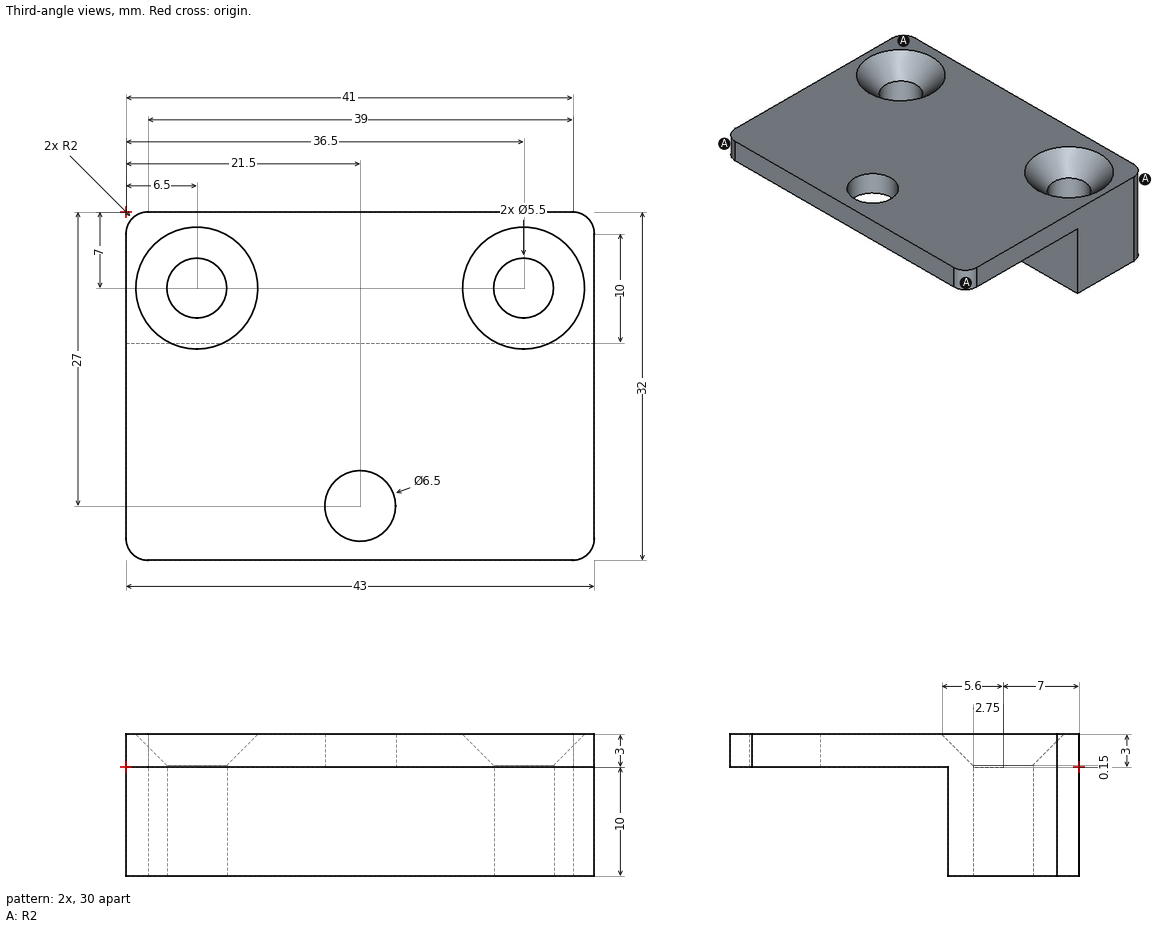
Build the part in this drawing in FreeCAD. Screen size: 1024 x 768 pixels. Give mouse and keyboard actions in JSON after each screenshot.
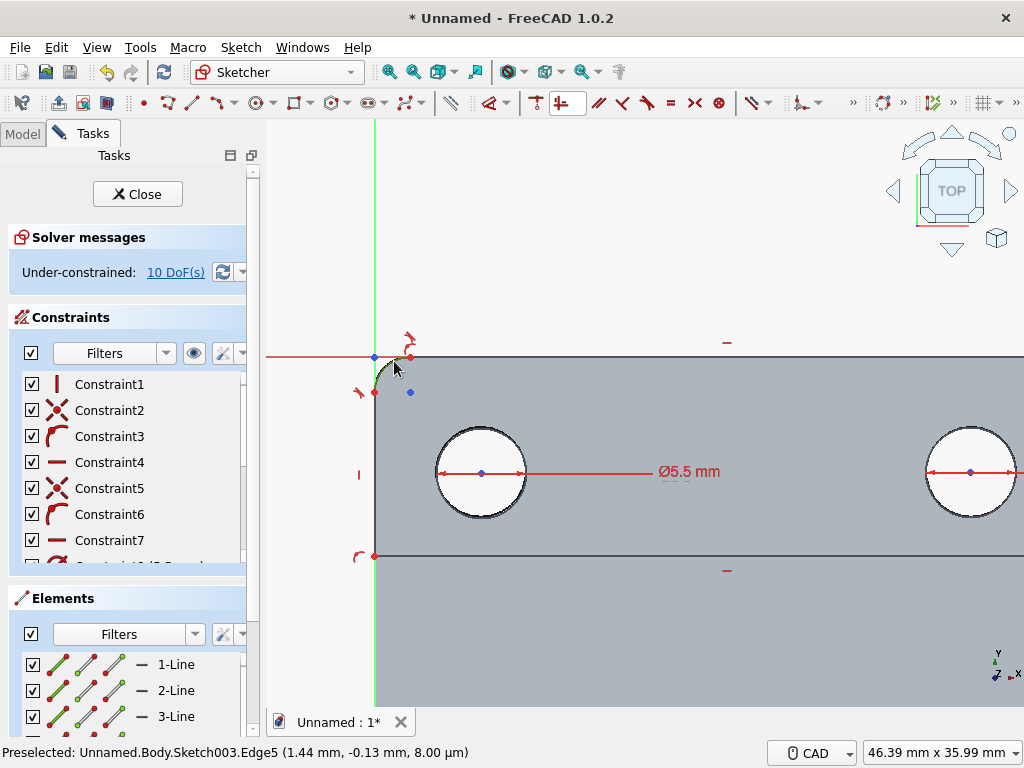
{"action": "scroll", "coordinate": [395, 361], "scroll_direction": "down", "scroll_amount": 3}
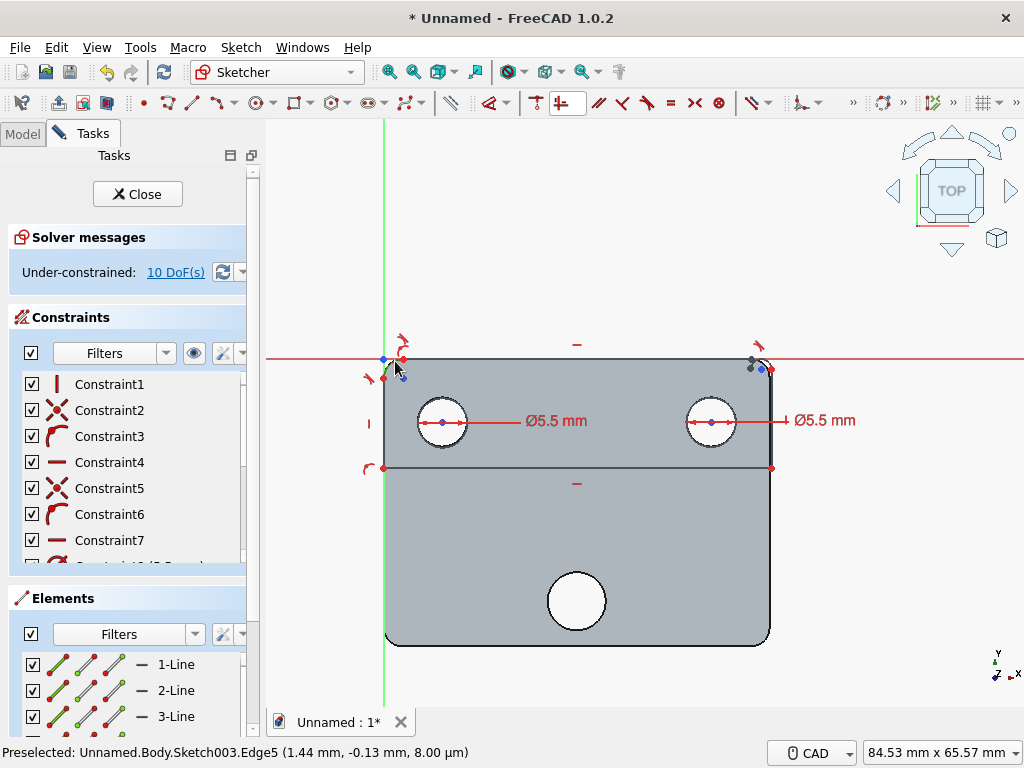
{"action": "scroll", "coordinate": [768, 361], "scroll_direction": "up", "scroll_amount": 2}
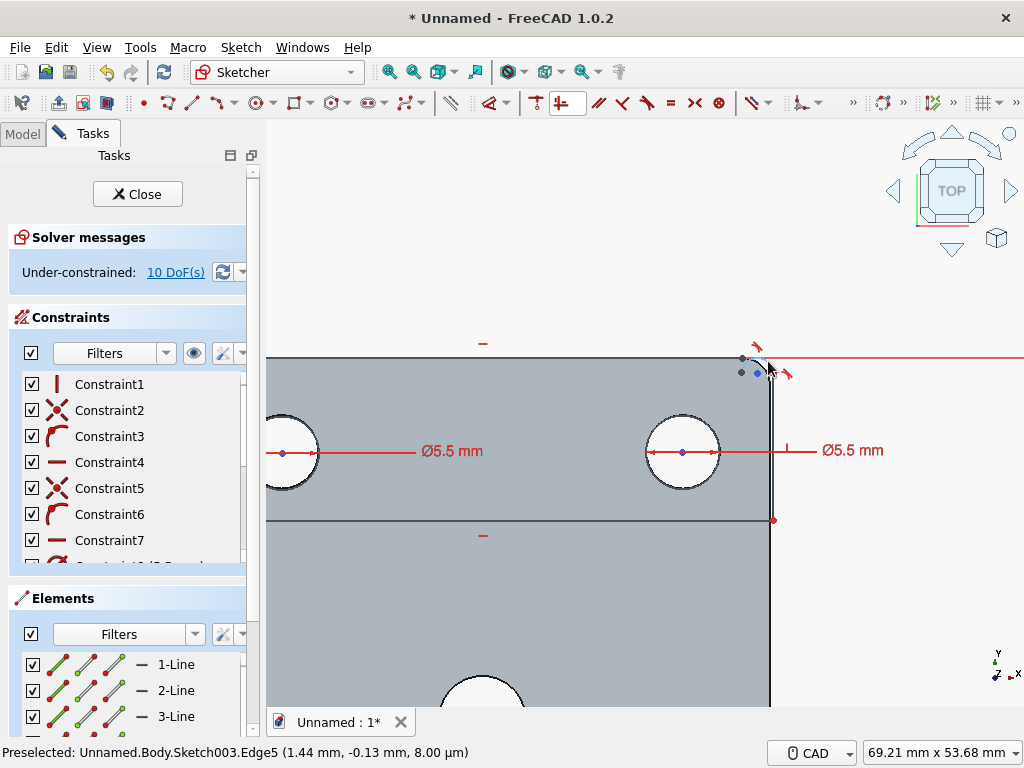
{"action": "left_click", "coordinate": [767, 361]}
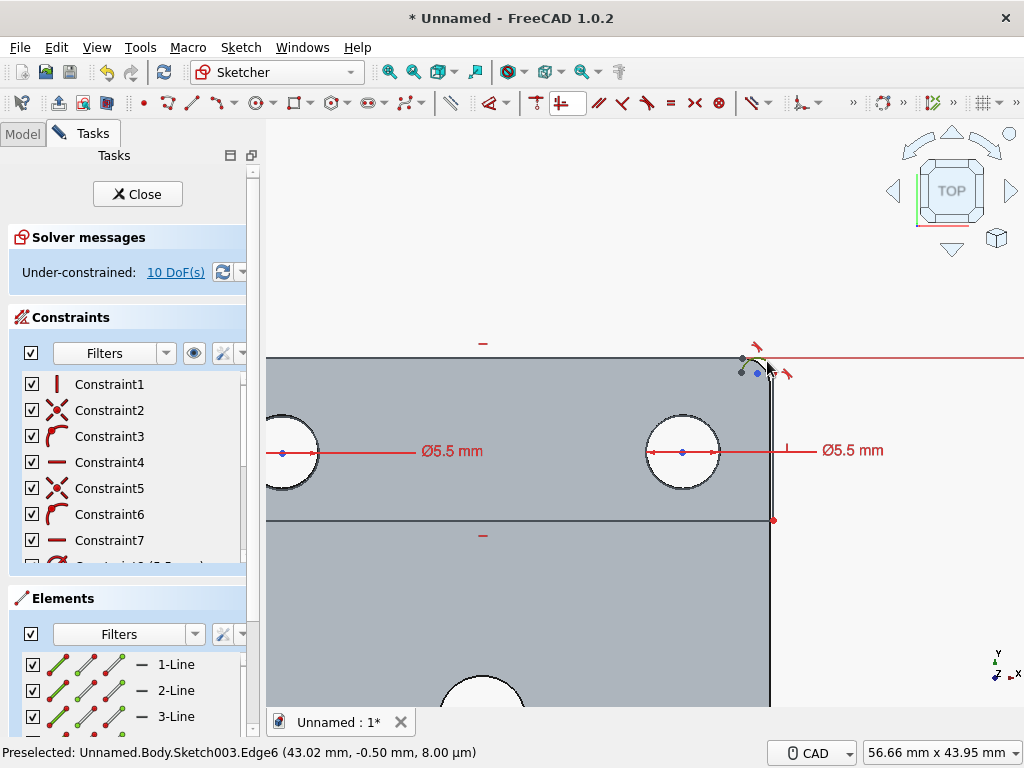
{"action": "key", "text": "e"}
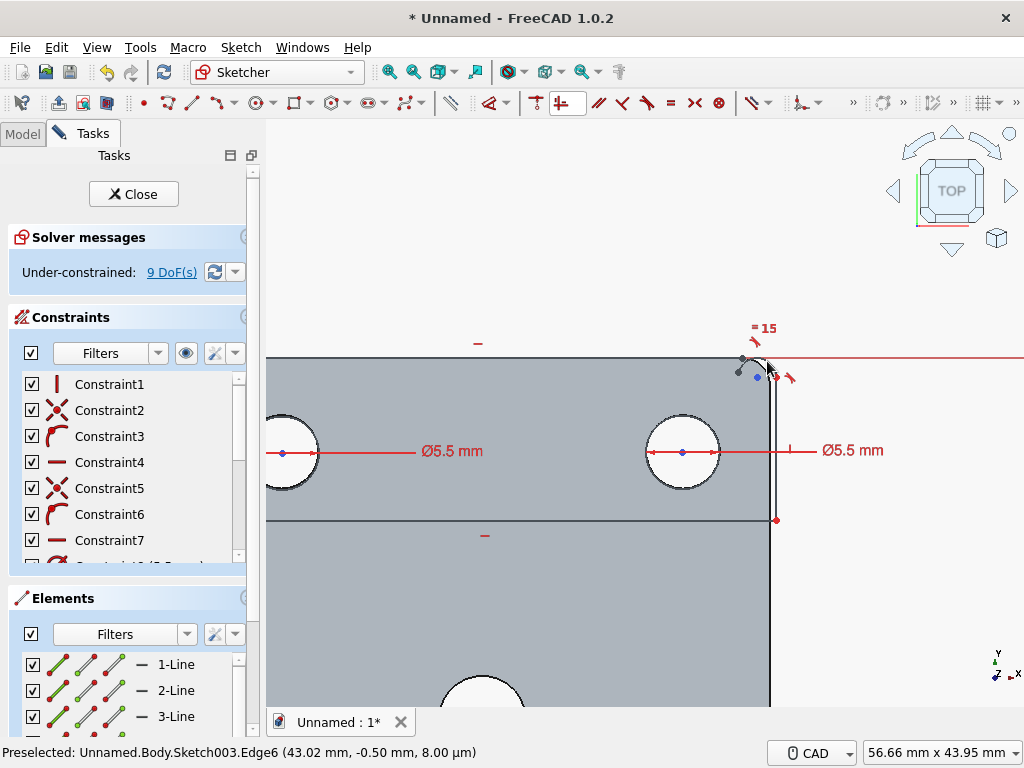
{"action": "key", "text": "d"}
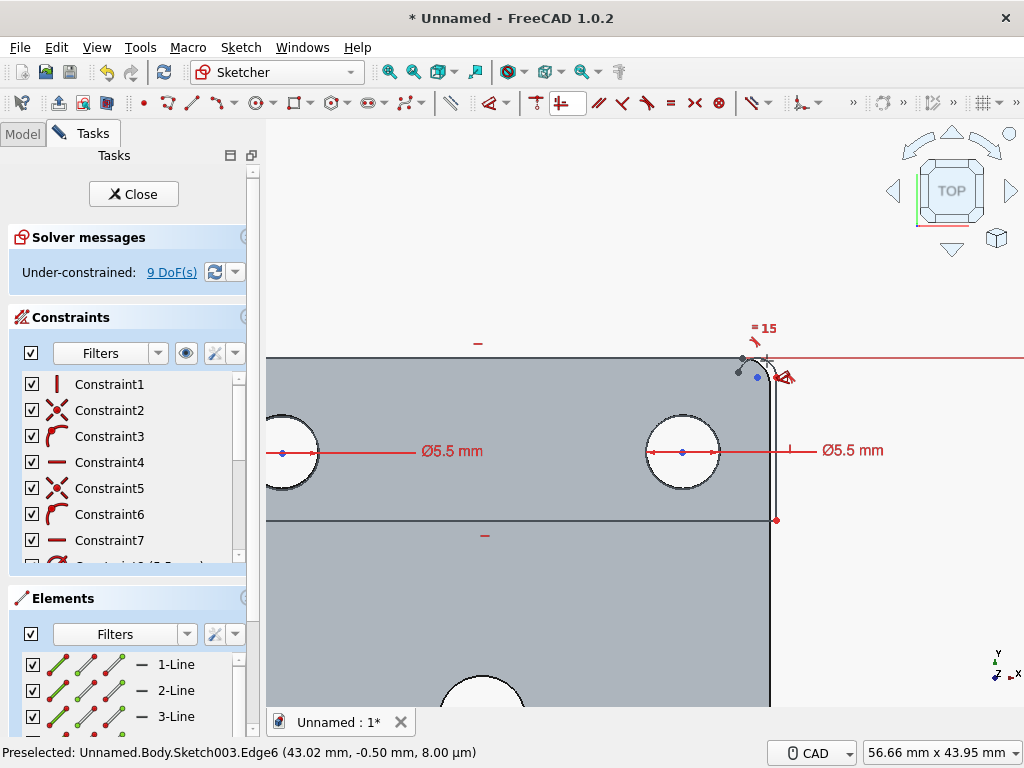
{"action": "scroll", "coordinate": [768, 361], "scroll_direction": "down", "scroll_amount": 2}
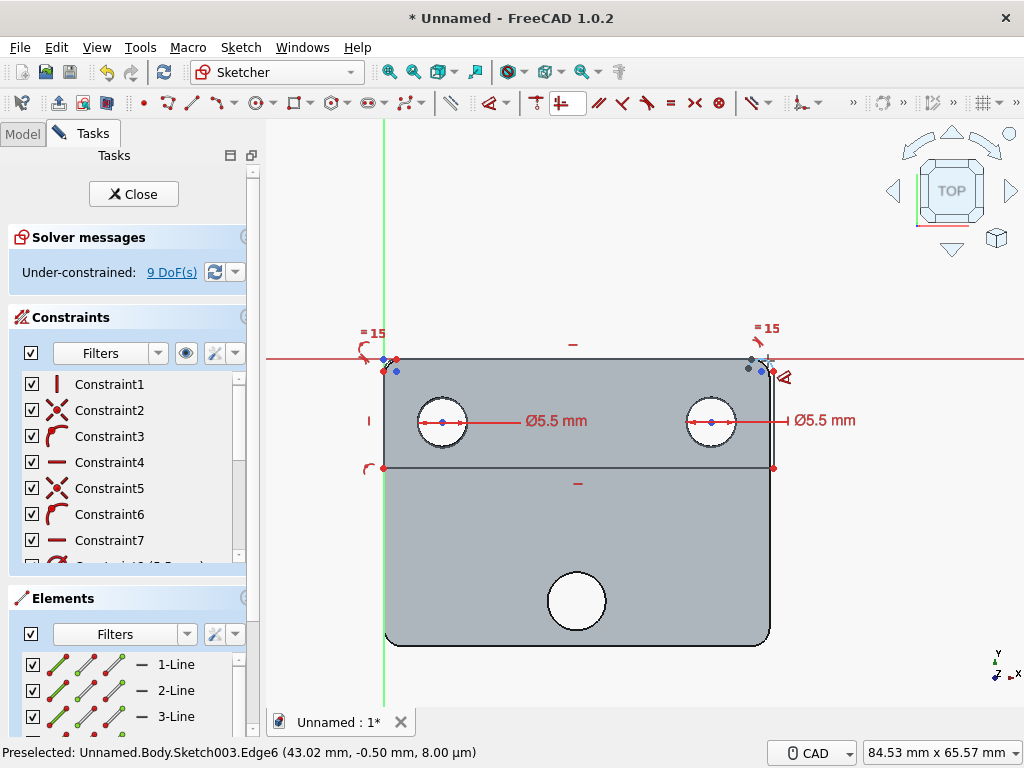
{"action": "scroll", "coordinate": [385, 366], "scroll_direction": "up", "scroll_amount": 5}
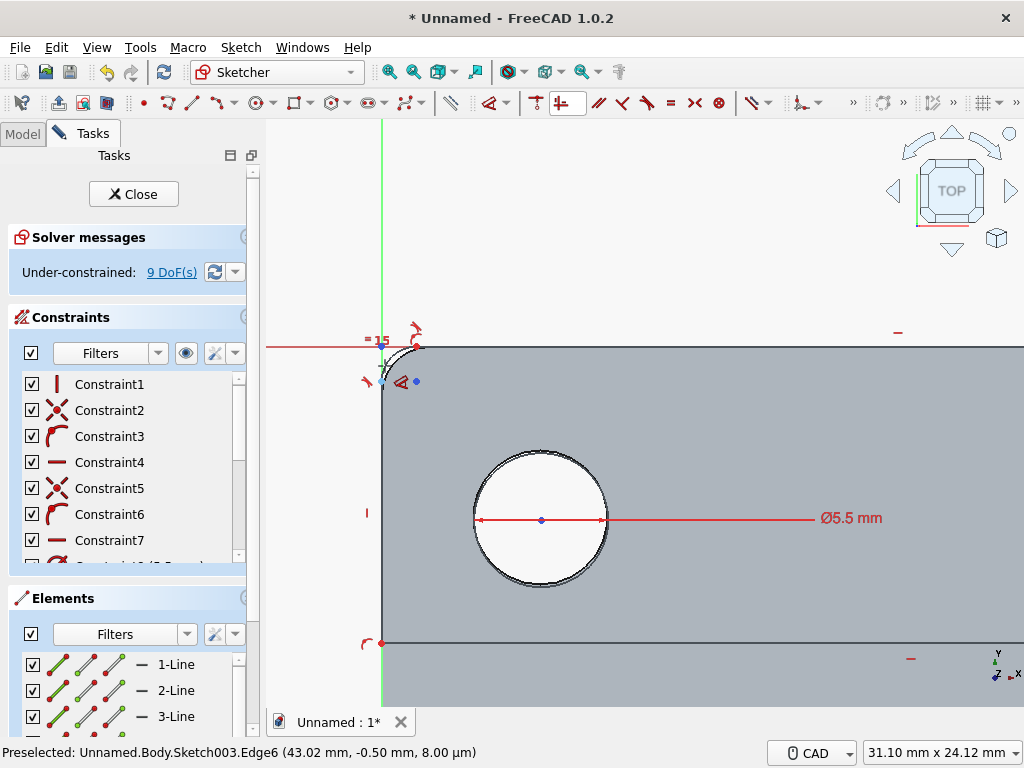
{"action": "left_click", "coordinate": [386, 366]}
{"action": "left_click", "coordinate": [350, 383]}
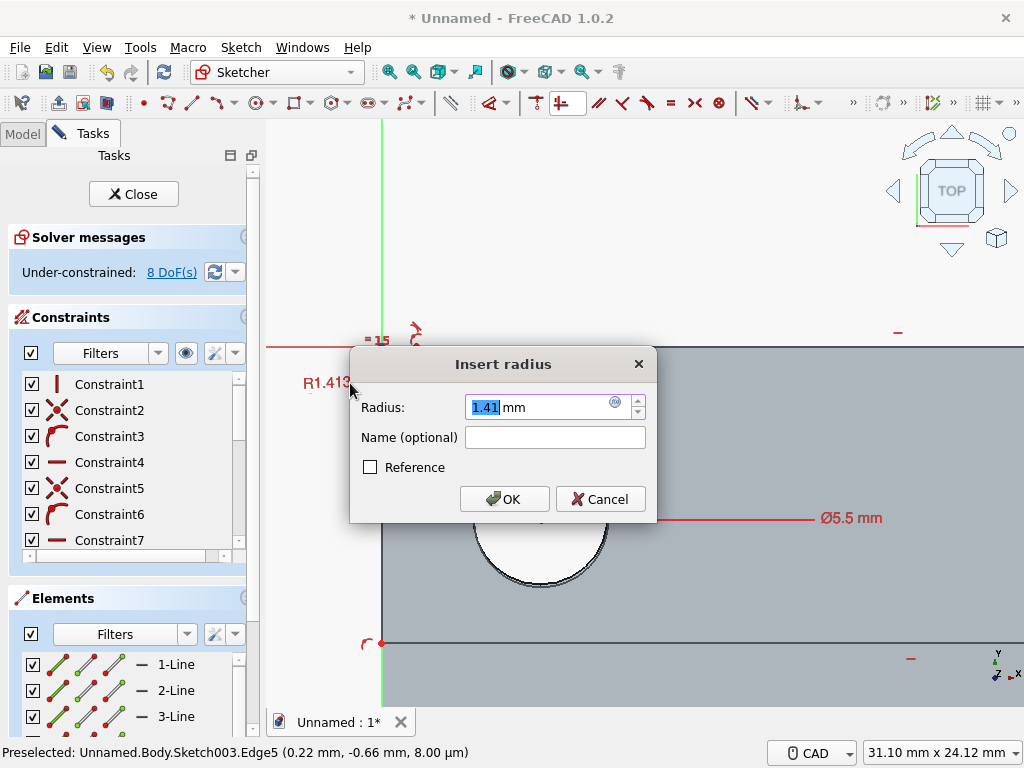
{"action": "type", "text": "2"}
{"action": "key", "text": "Return"}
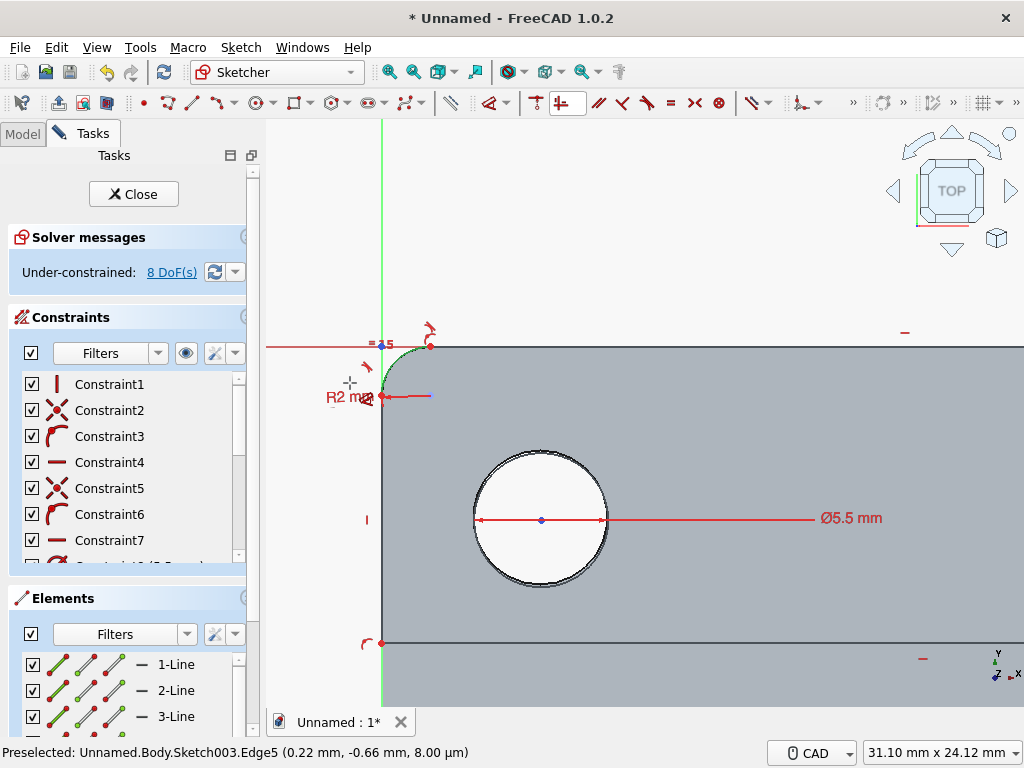
{"action": "scroll", "coordinate": [385, 366], "scroll_direction": "down", "scroll_amount": 5}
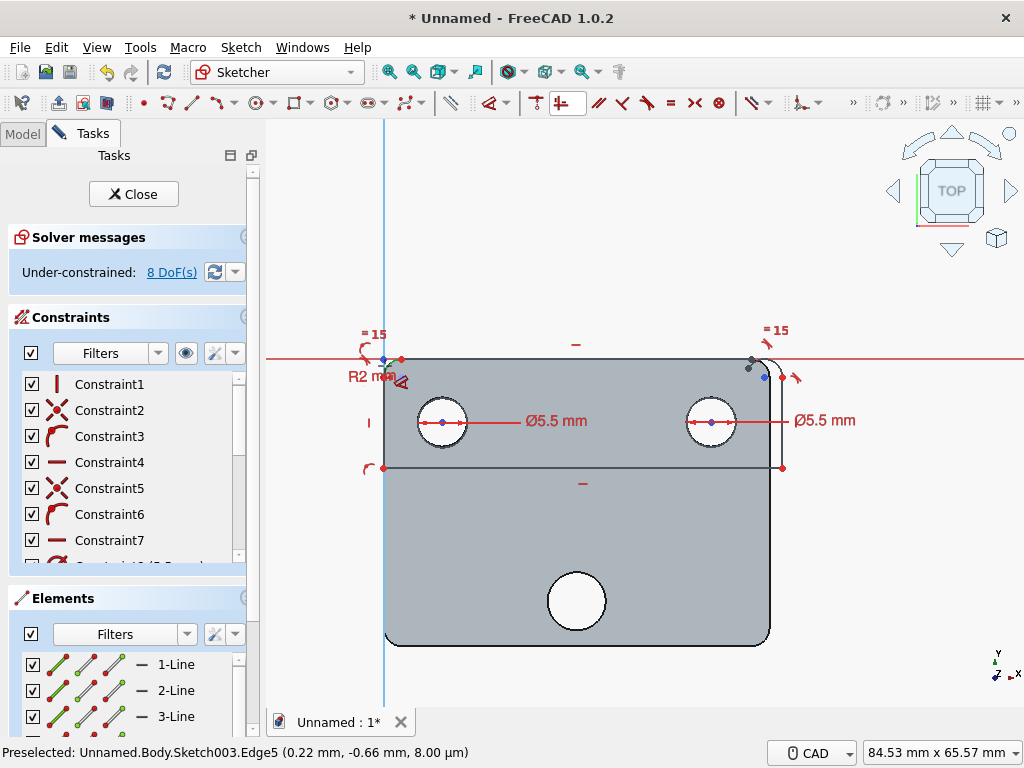
{"action": "left_click", "coordinate": [711, 422]}
{"action": "left_click", "coordinate": [350, 405]}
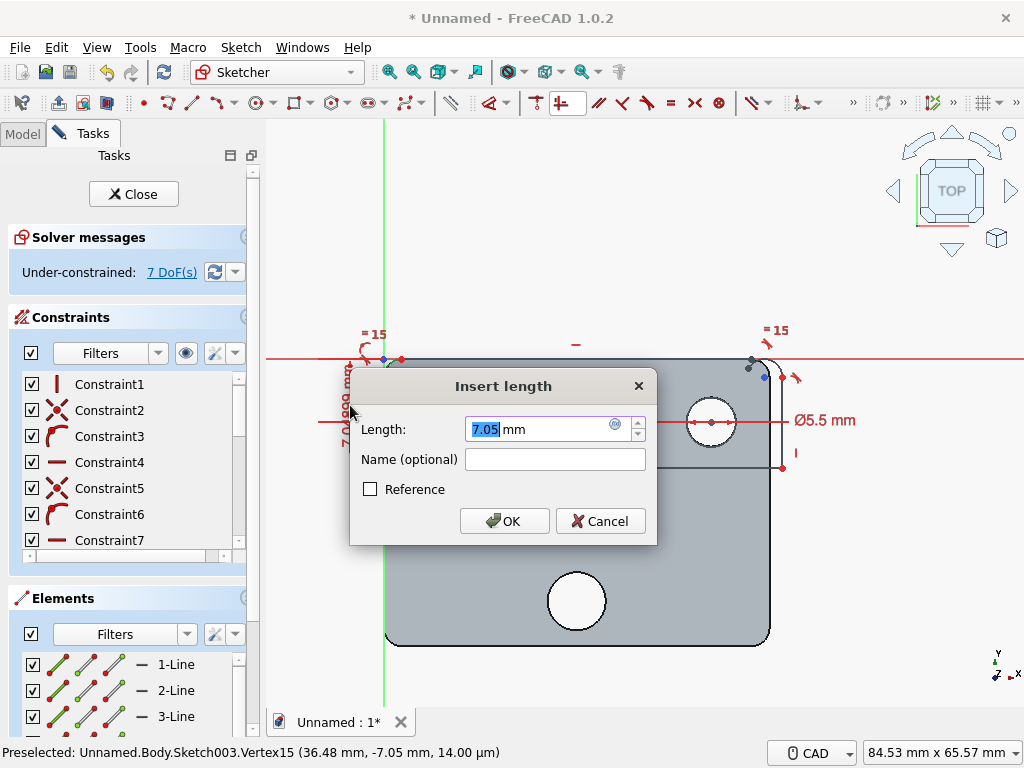
{"action": "type", "text": "7"}
{"action": "key", "text": "Return"}